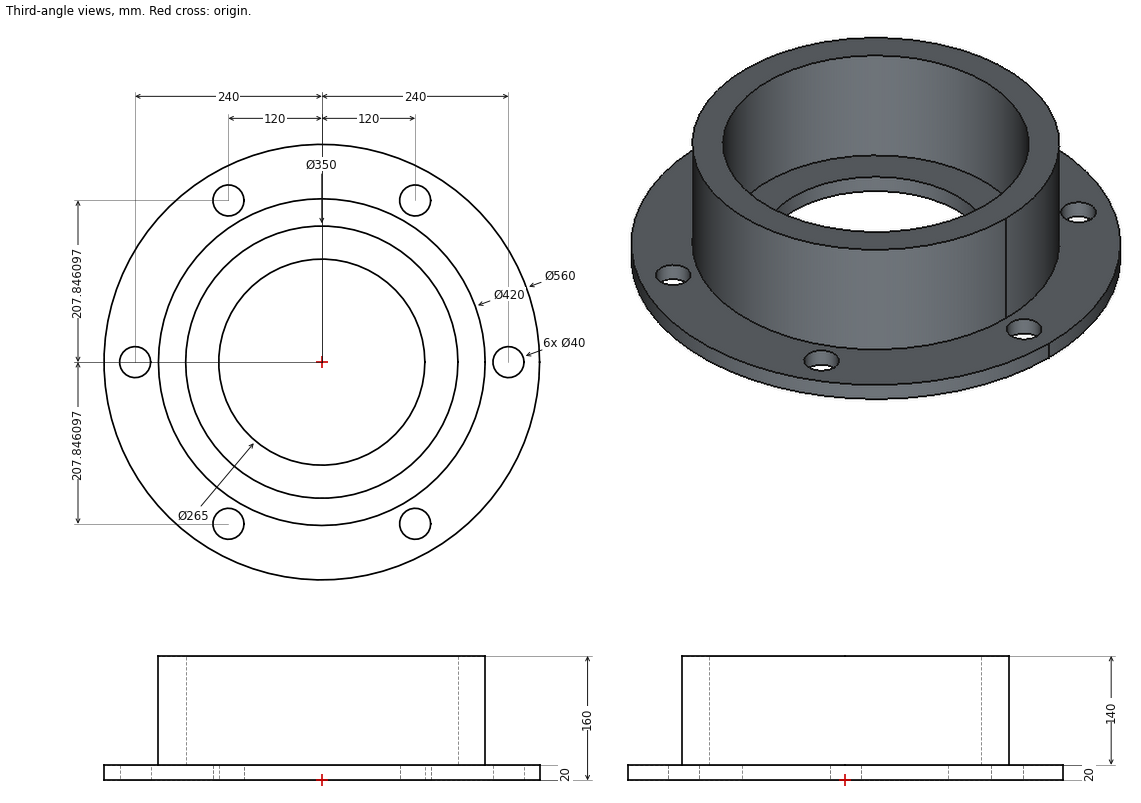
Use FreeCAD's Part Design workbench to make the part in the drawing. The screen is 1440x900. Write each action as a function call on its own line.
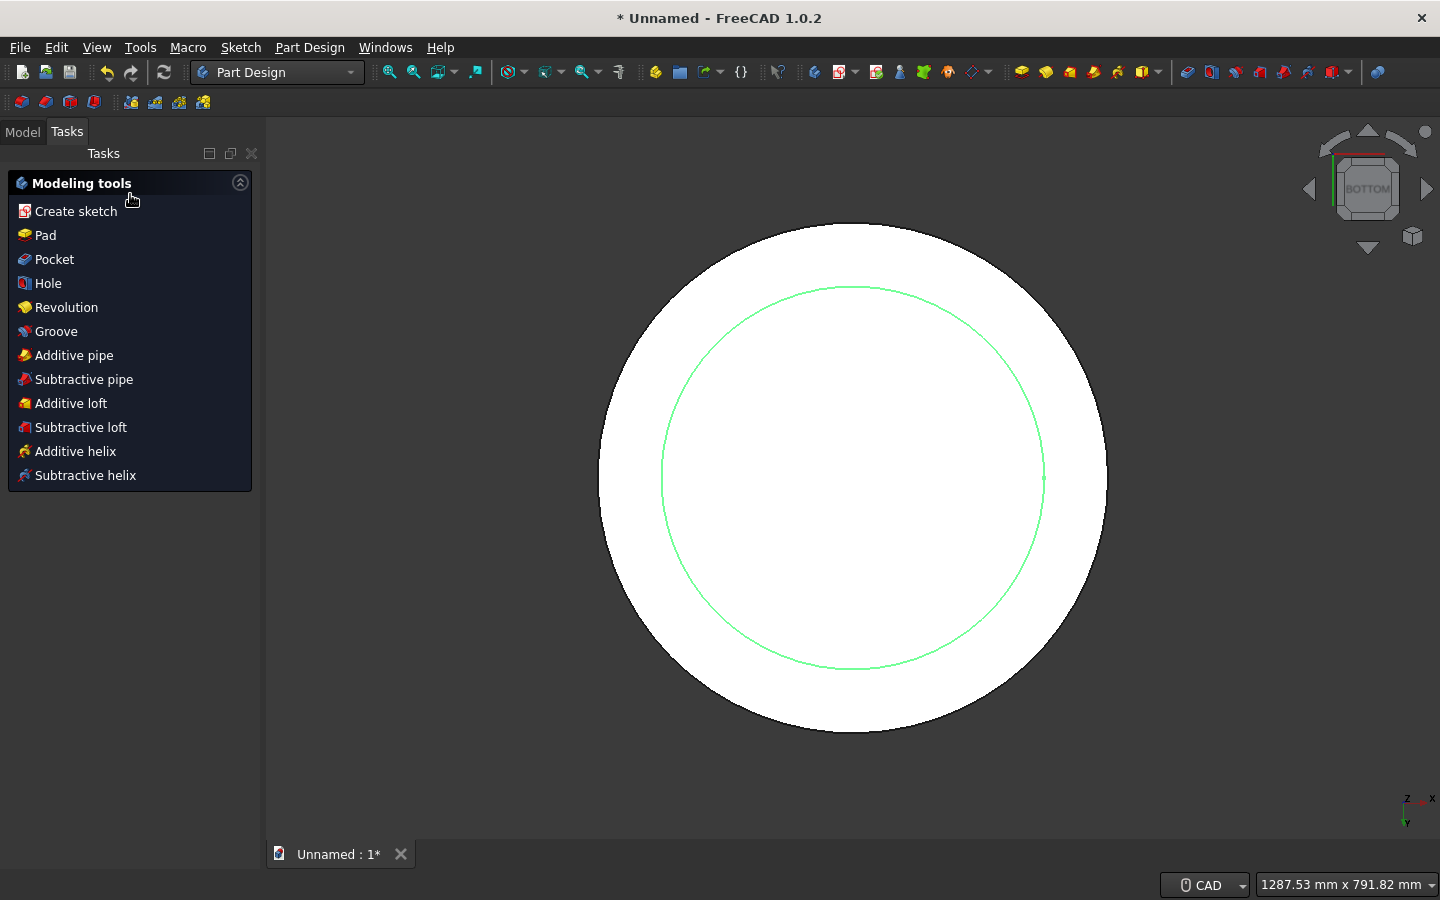
click(1022, 72)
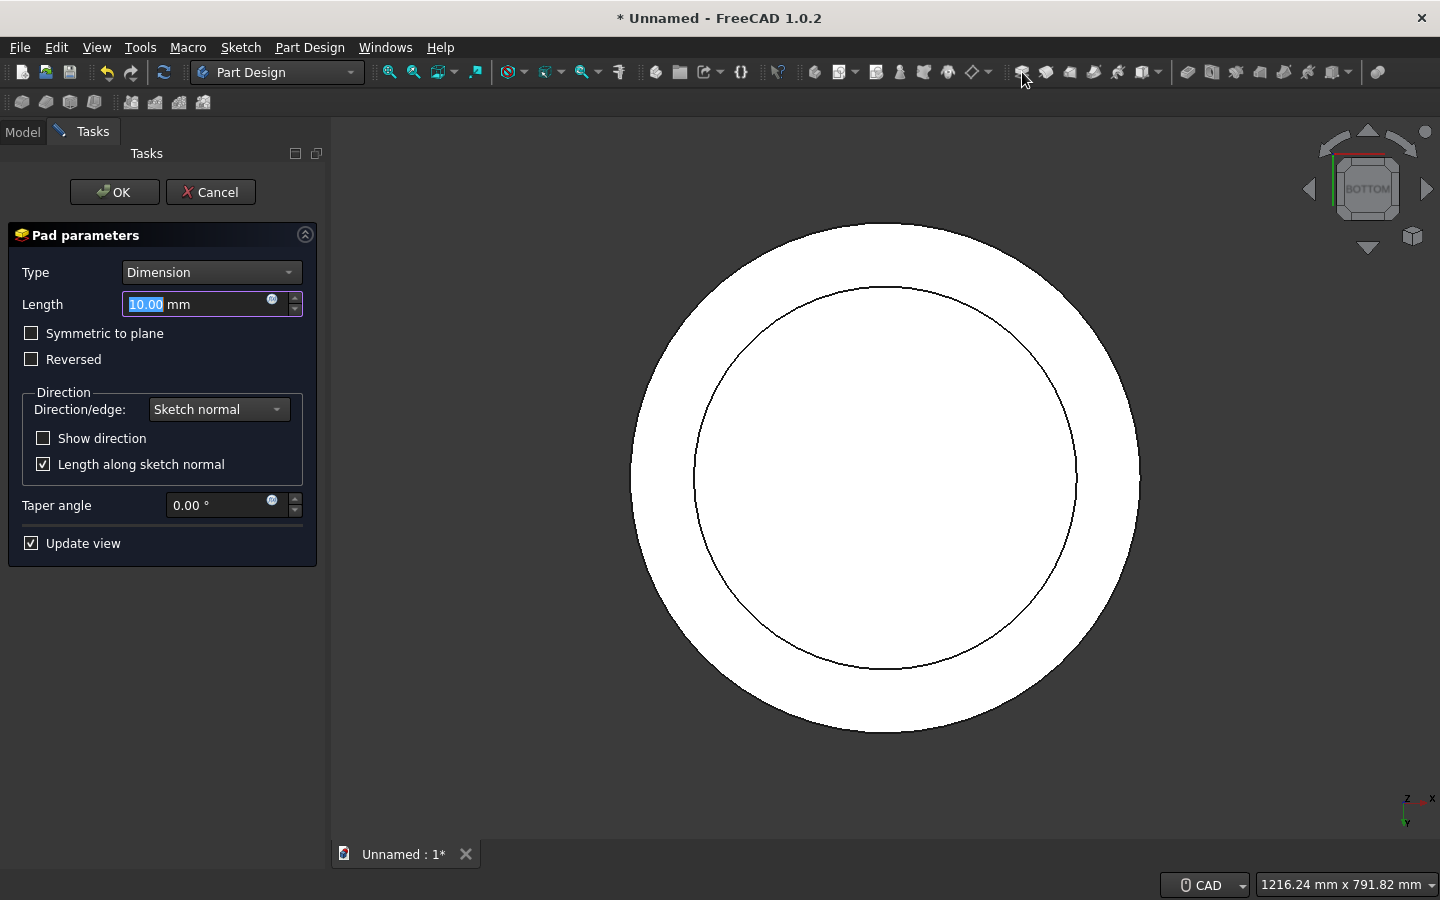
text(160)
key(Tab)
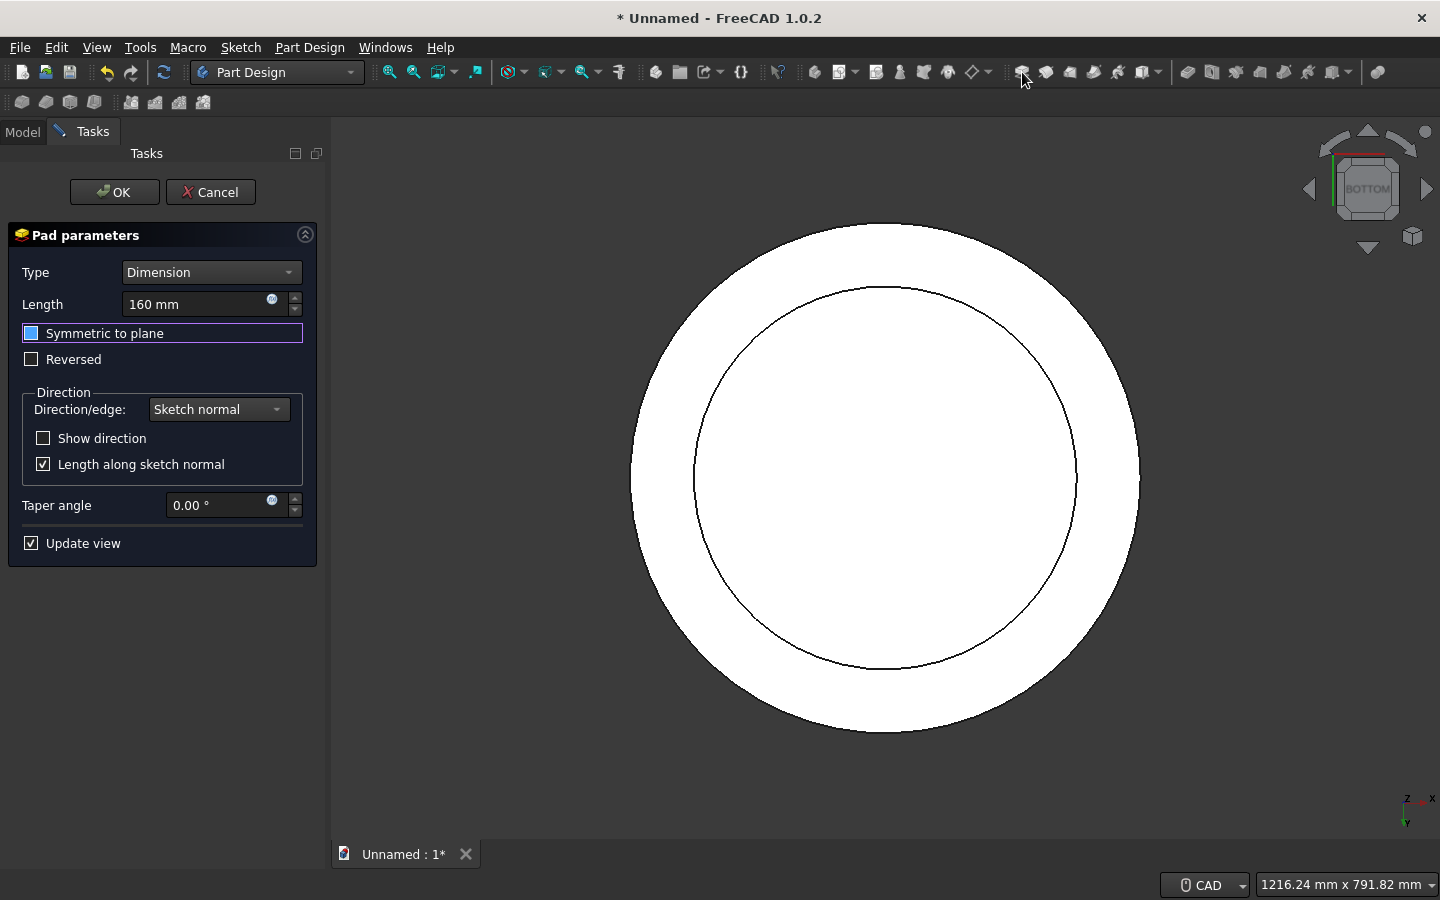
click(30, 359)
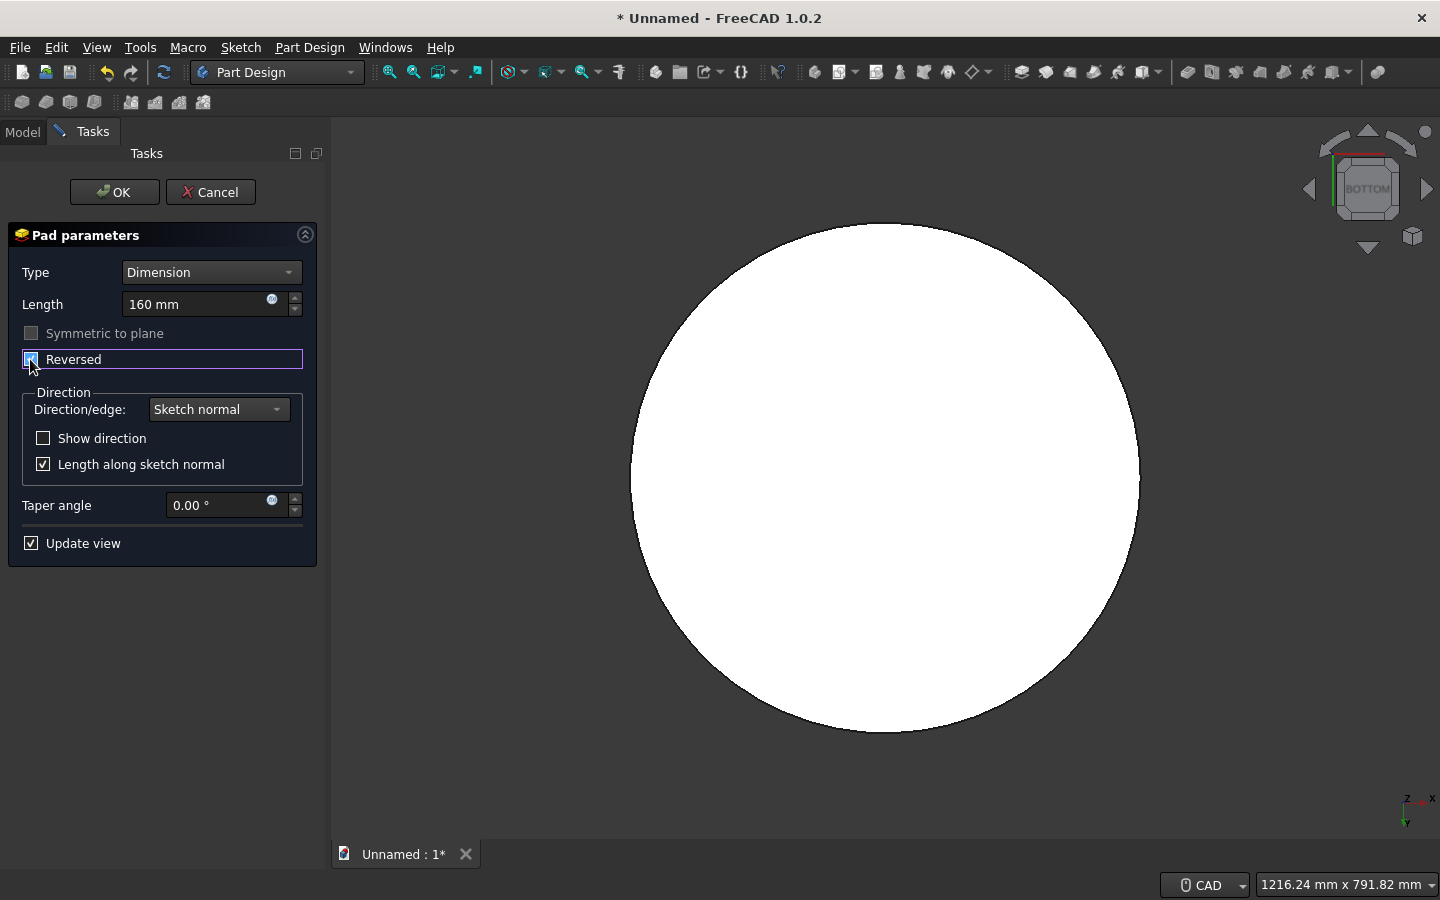
click(115, 192)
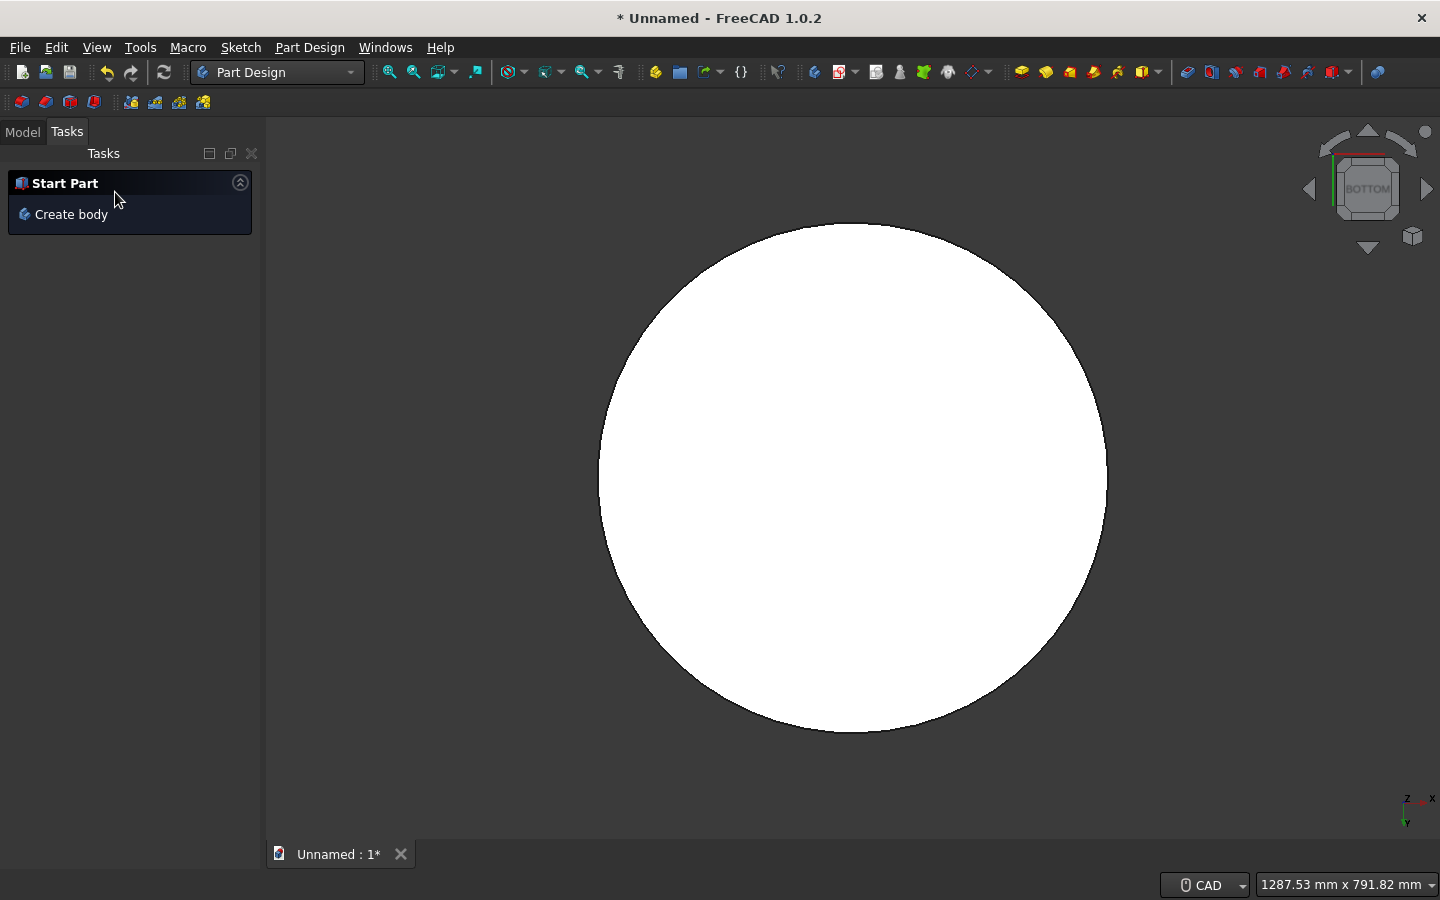
key(0)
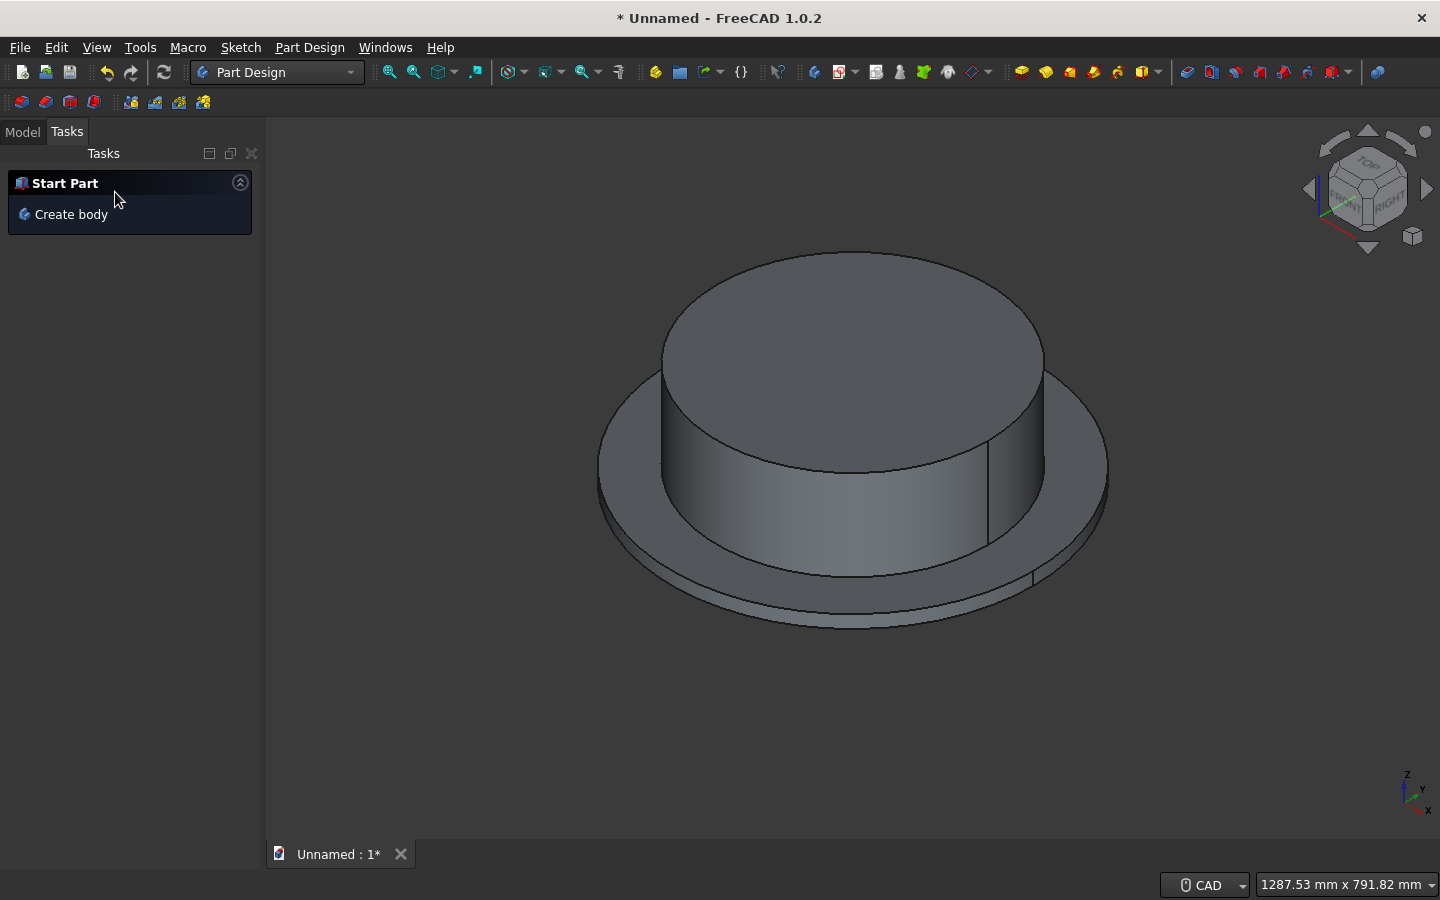
click(853, 362)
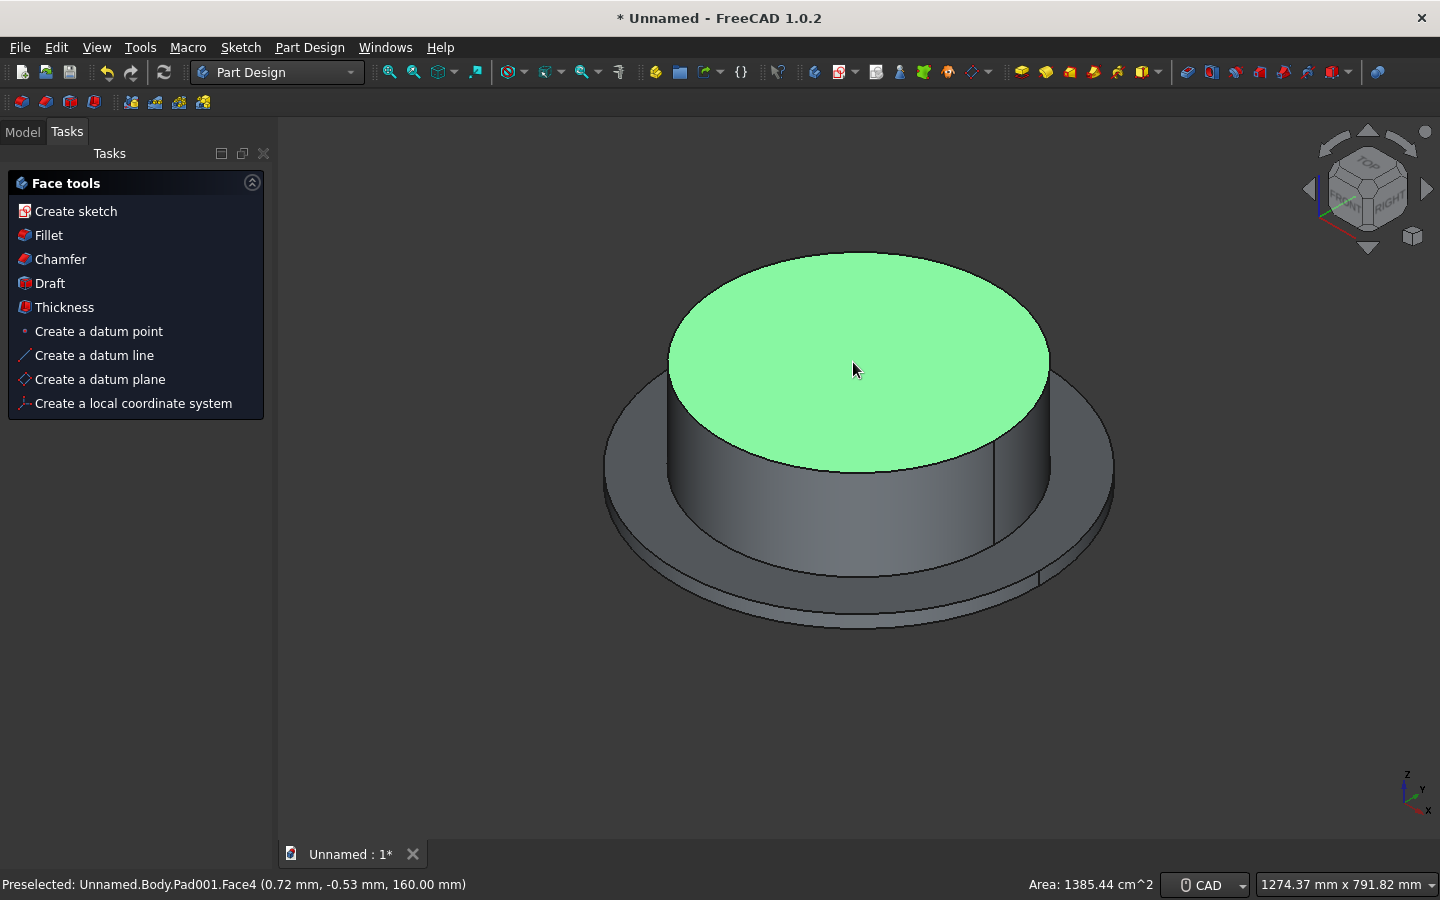
click(840, 72)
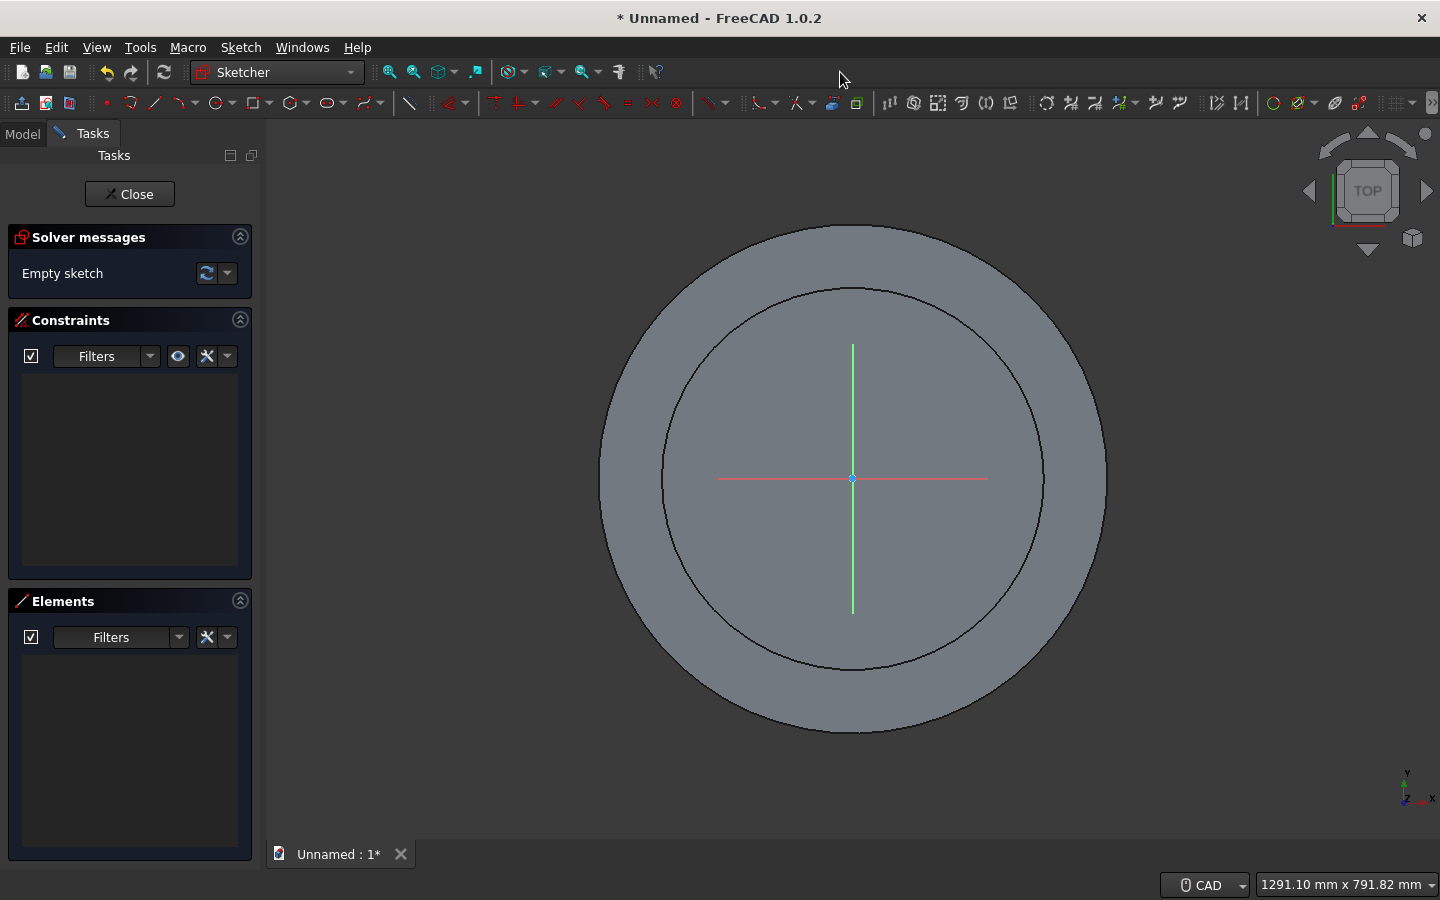
scroll(992, 479, up, 2)